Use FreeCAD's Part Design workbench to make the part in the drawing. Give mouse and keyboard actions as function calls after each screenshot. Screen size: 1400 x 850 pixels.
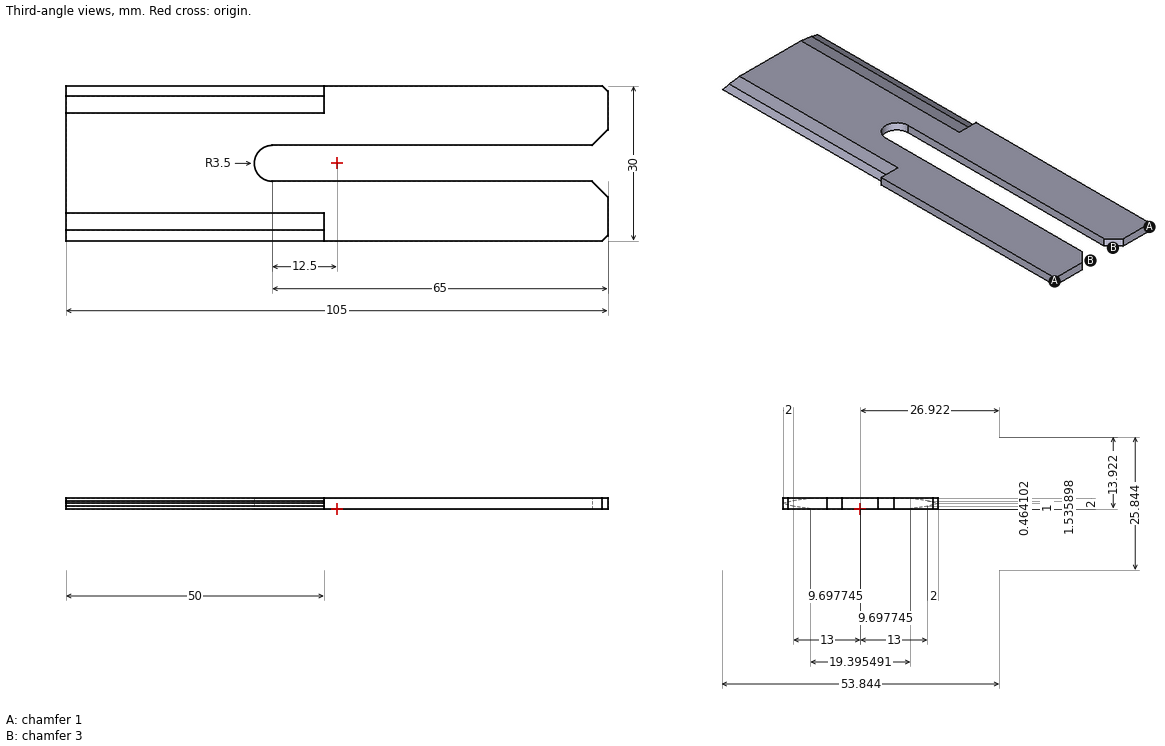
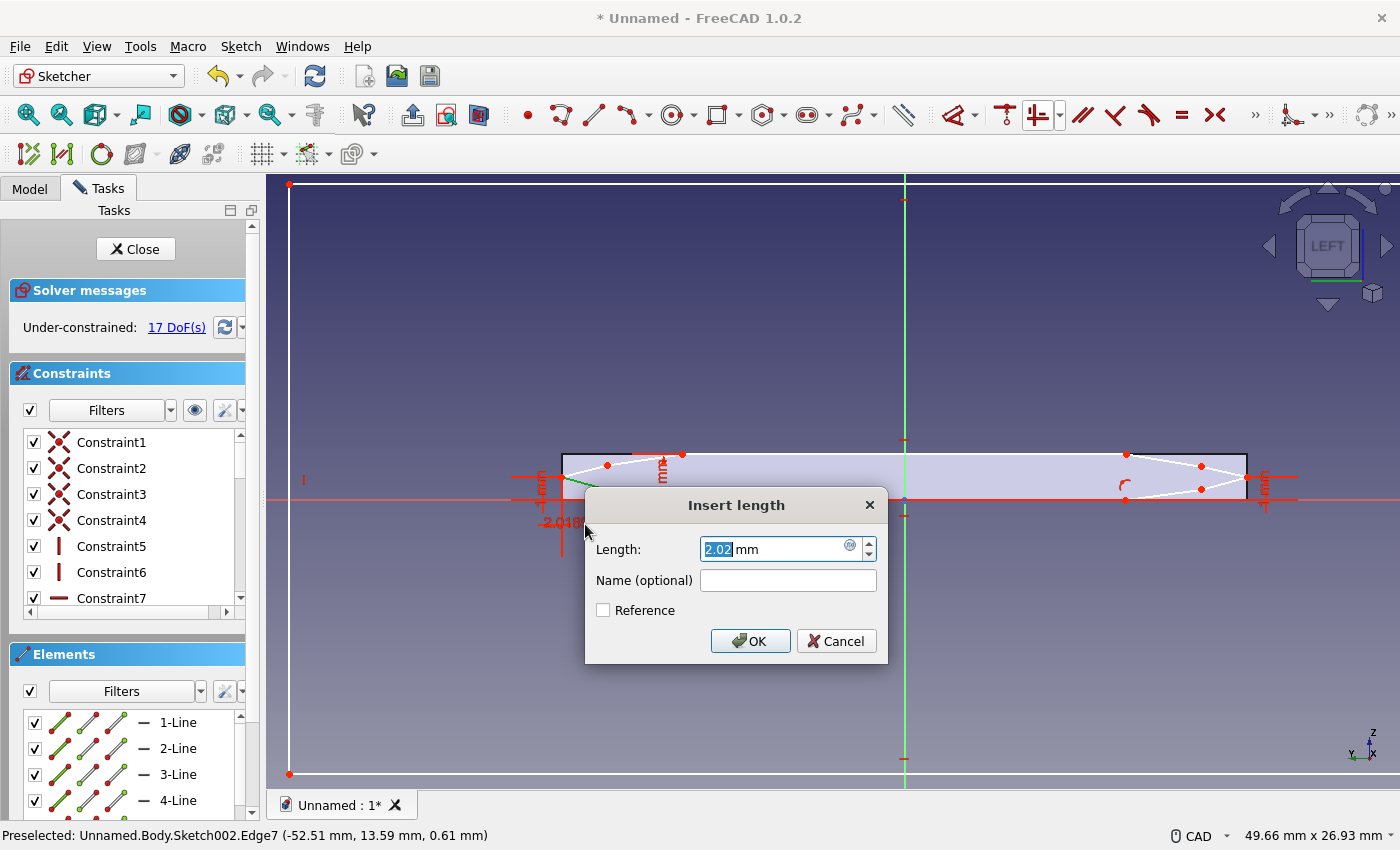
text(2)
key(Return)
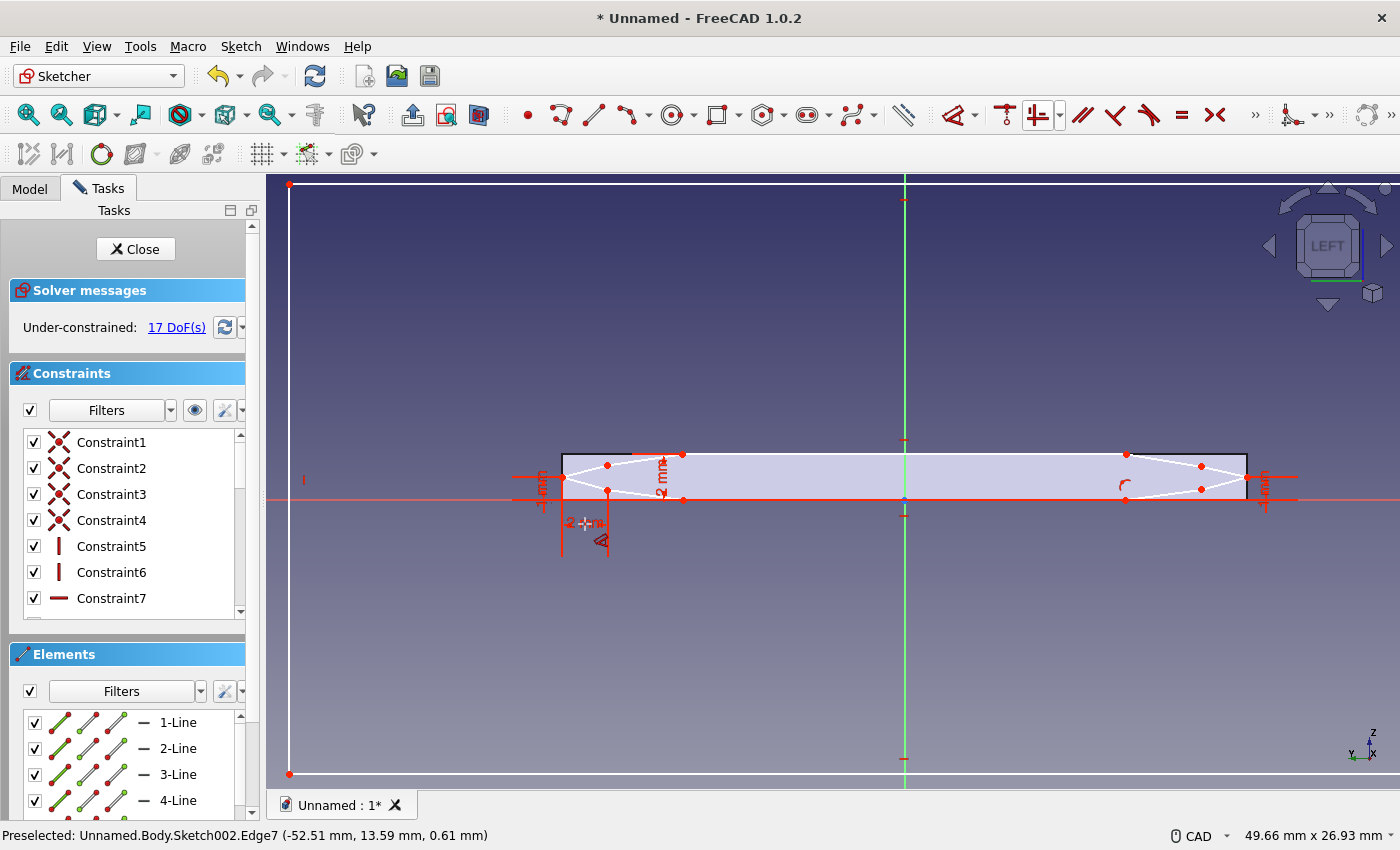
click(594, 469)
click(585, 431)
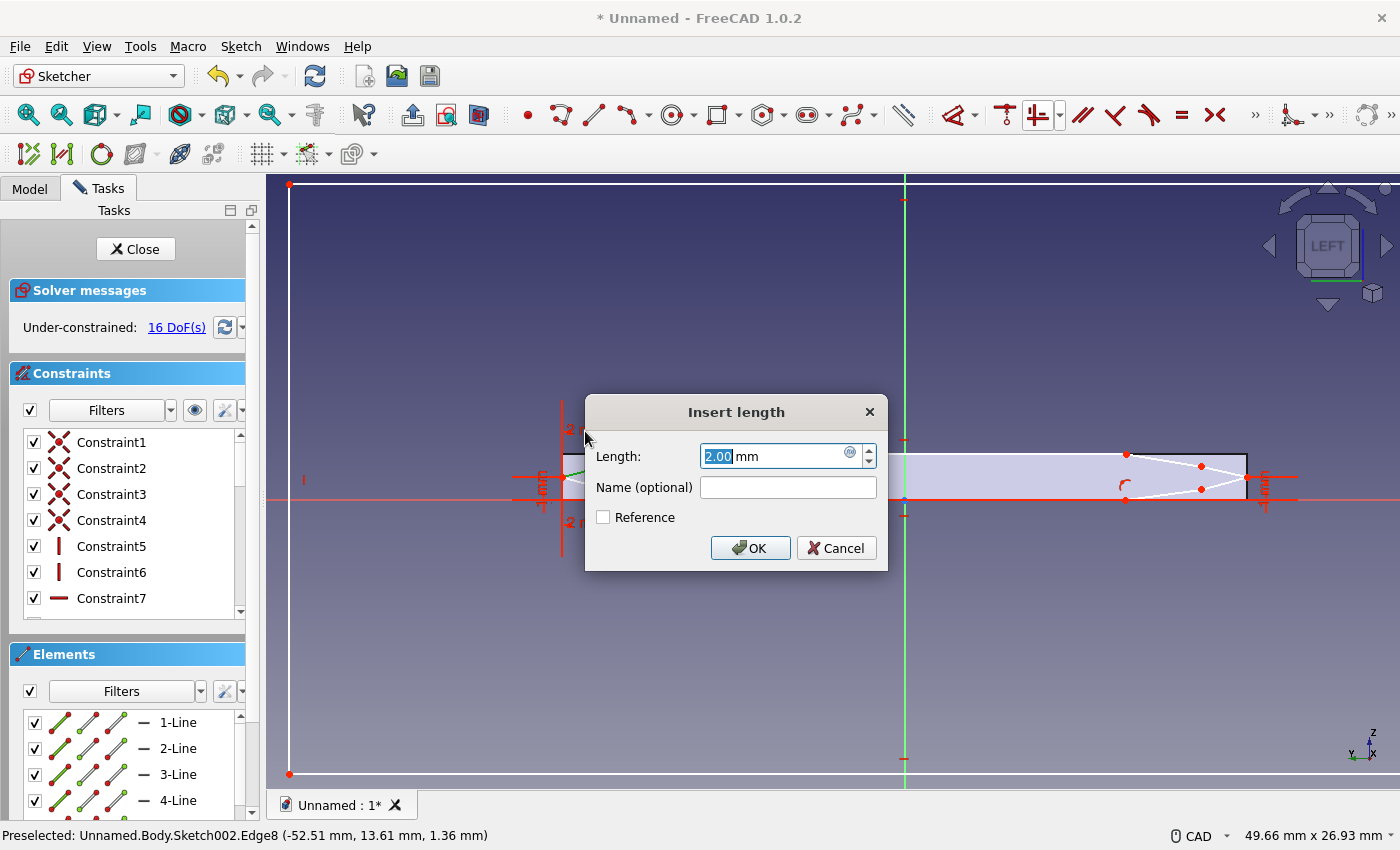
text(2)
key(Return)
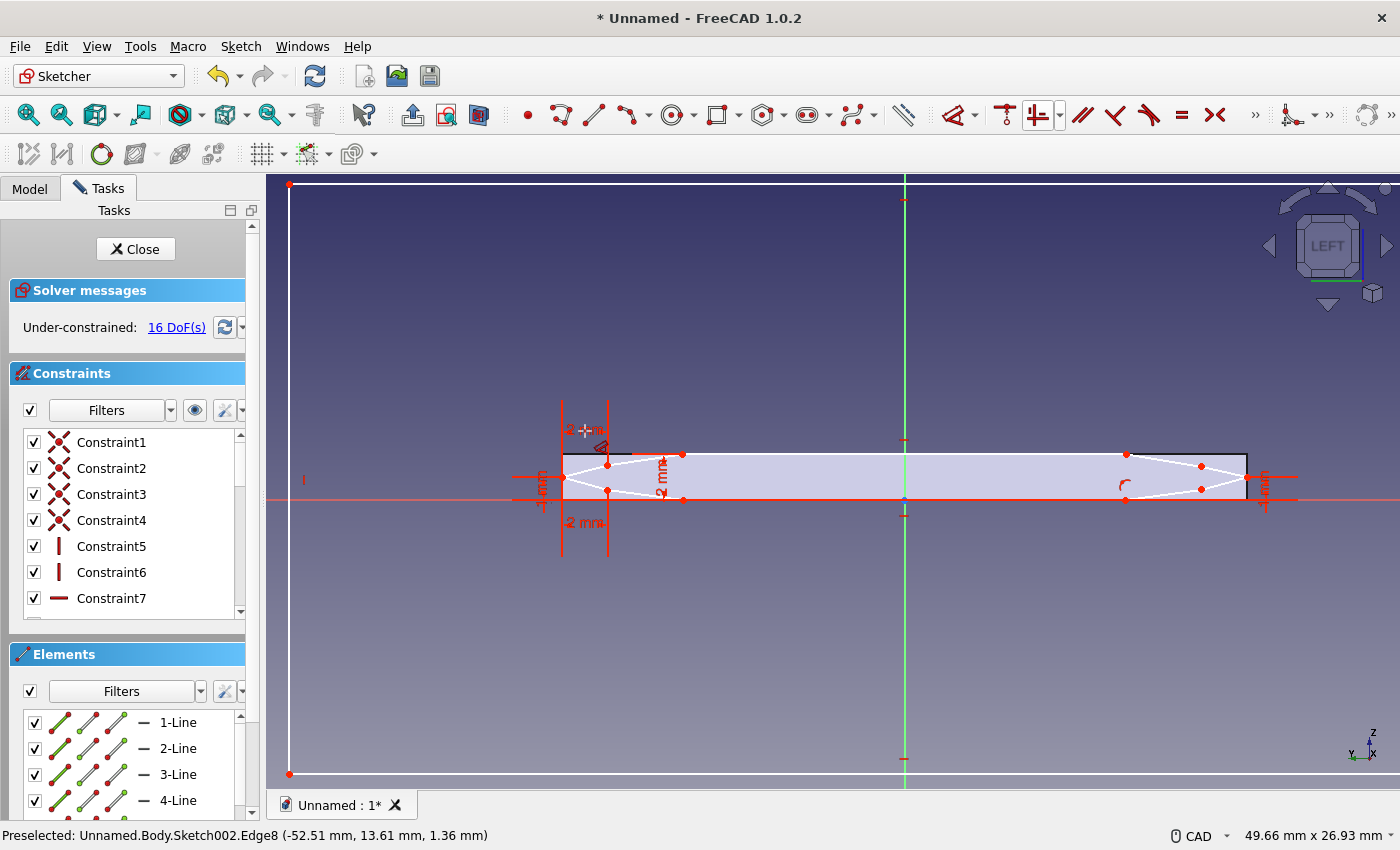
click(1215, 470)
click(1218, 433)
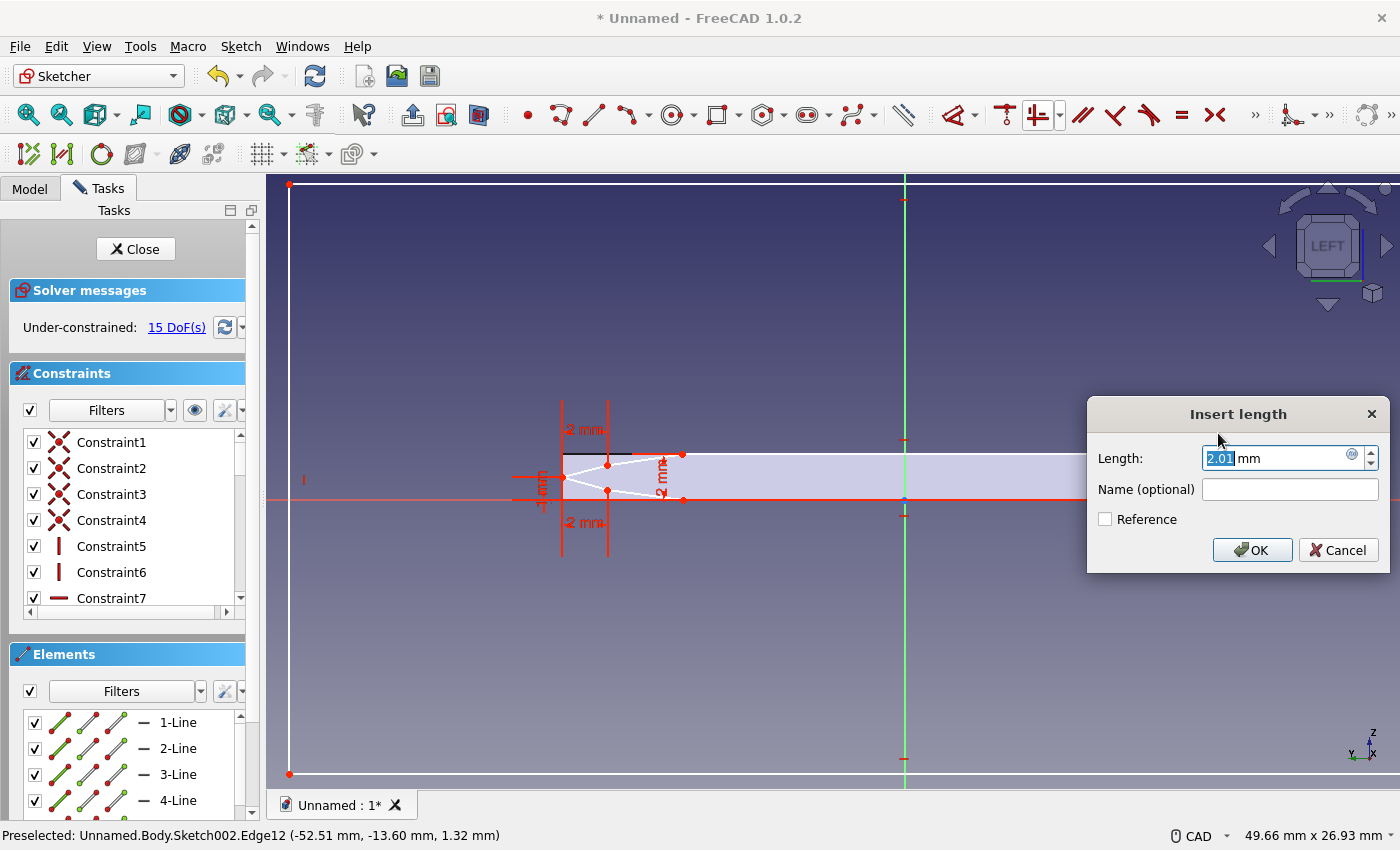
text(2)
key(Return)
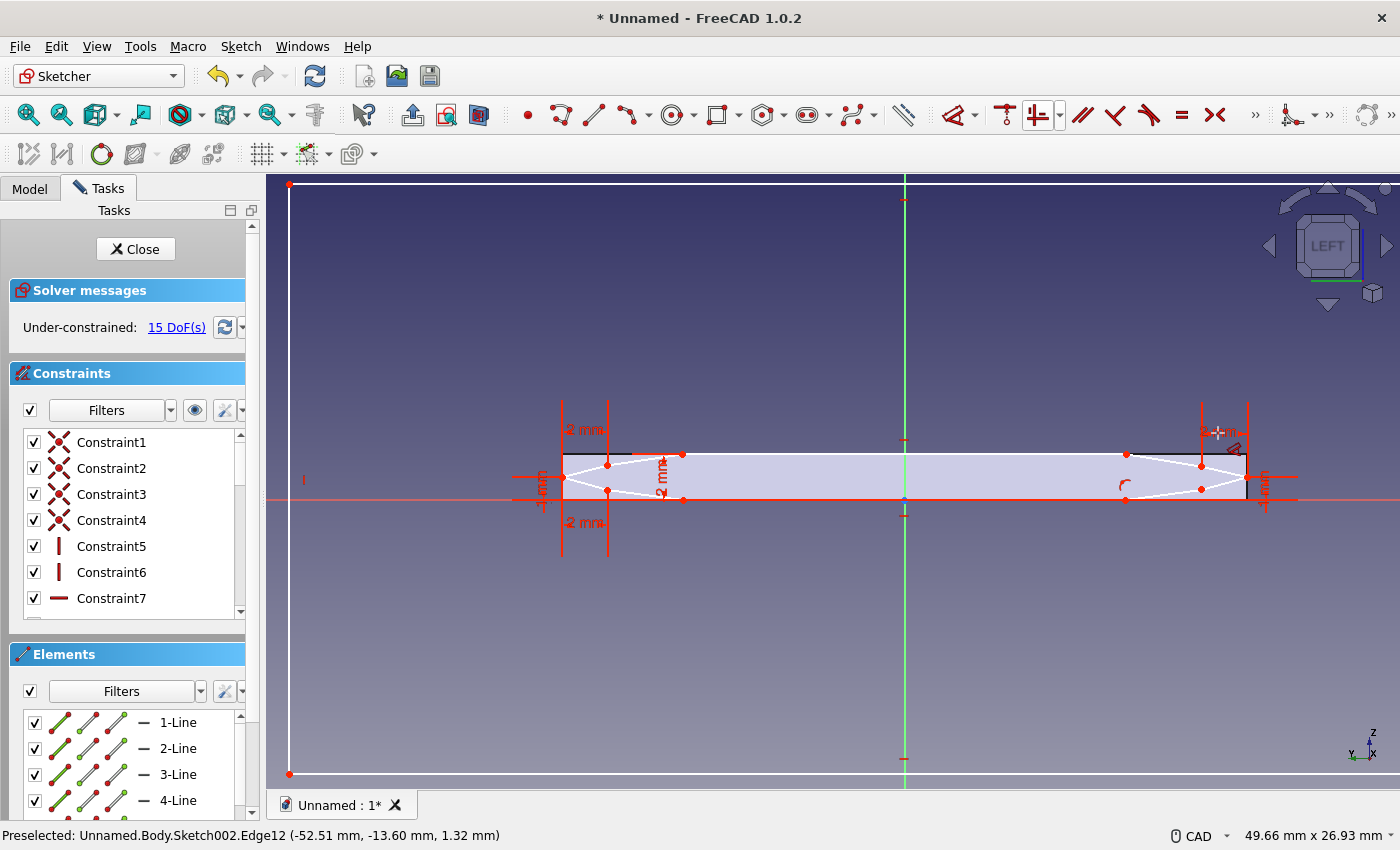
click(1215, 486)
click(1218, 524)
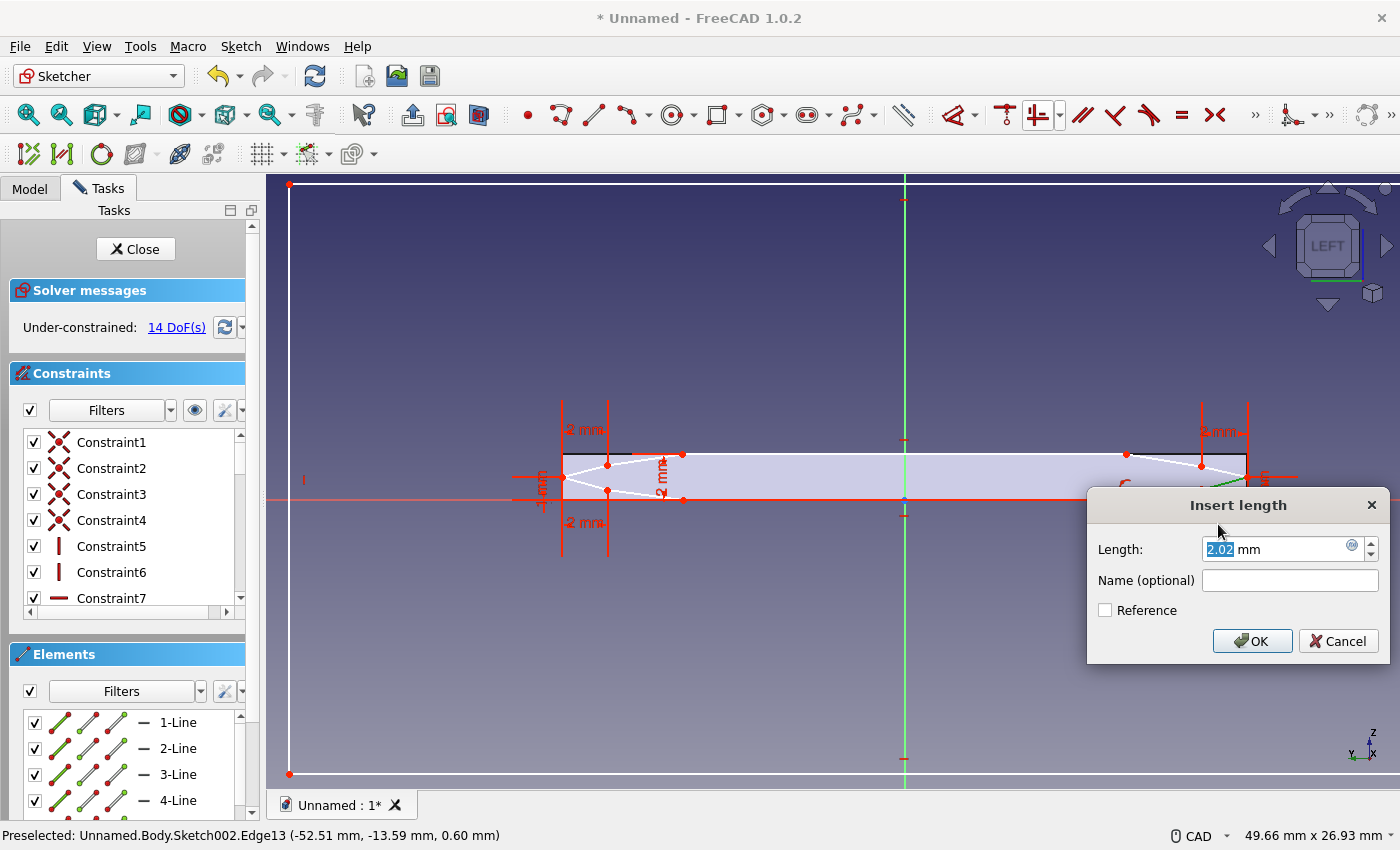
text(2)
key(Return)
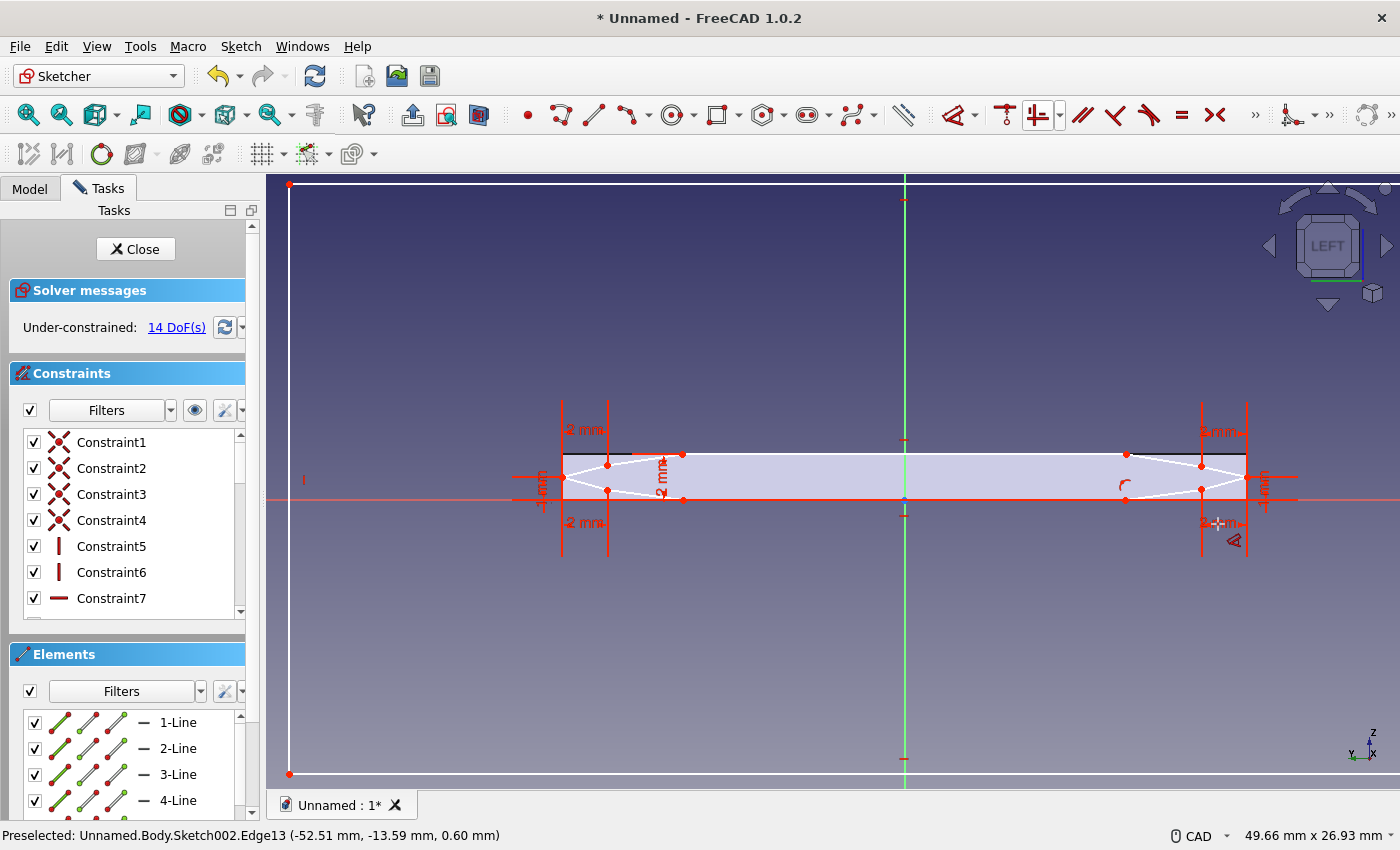
click(608, 490)
click(756, 534)